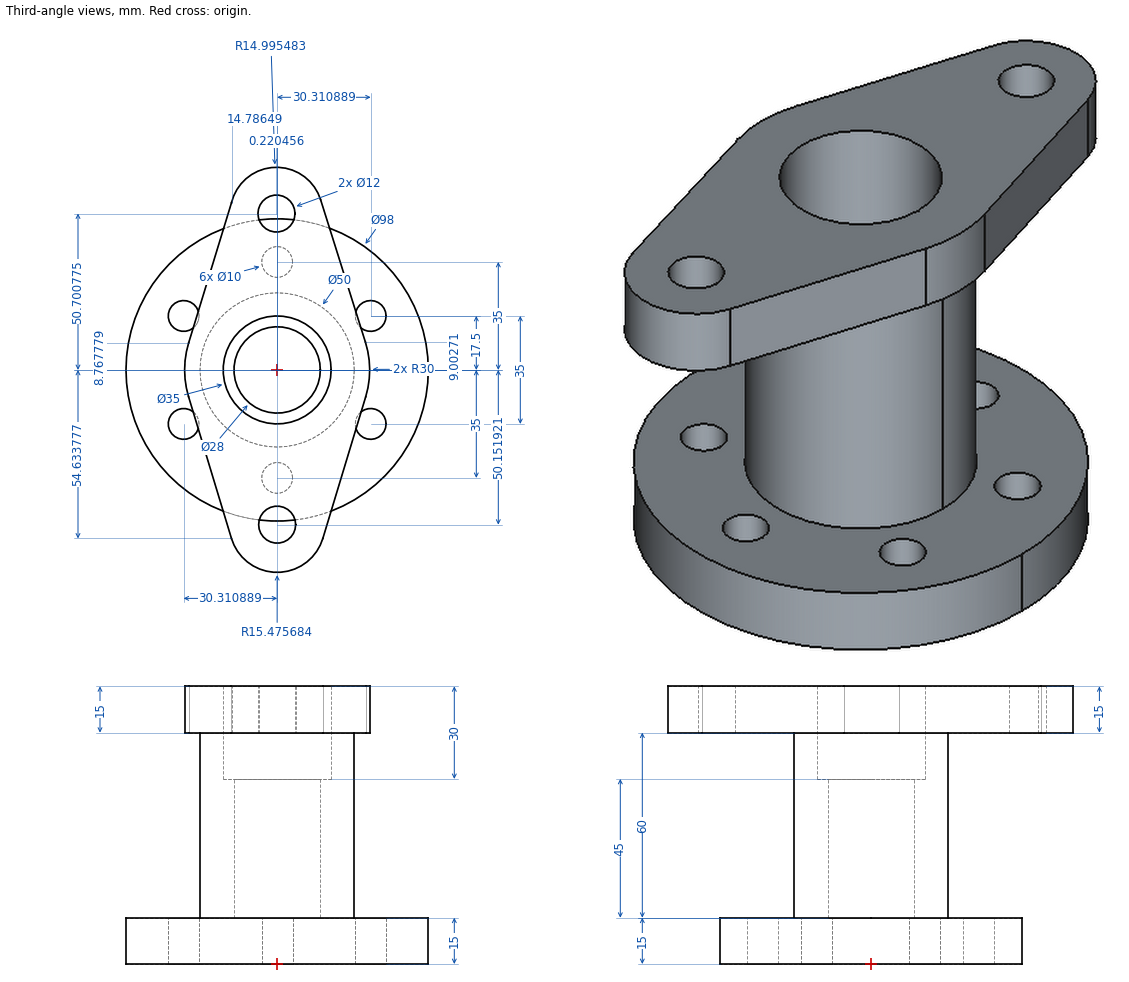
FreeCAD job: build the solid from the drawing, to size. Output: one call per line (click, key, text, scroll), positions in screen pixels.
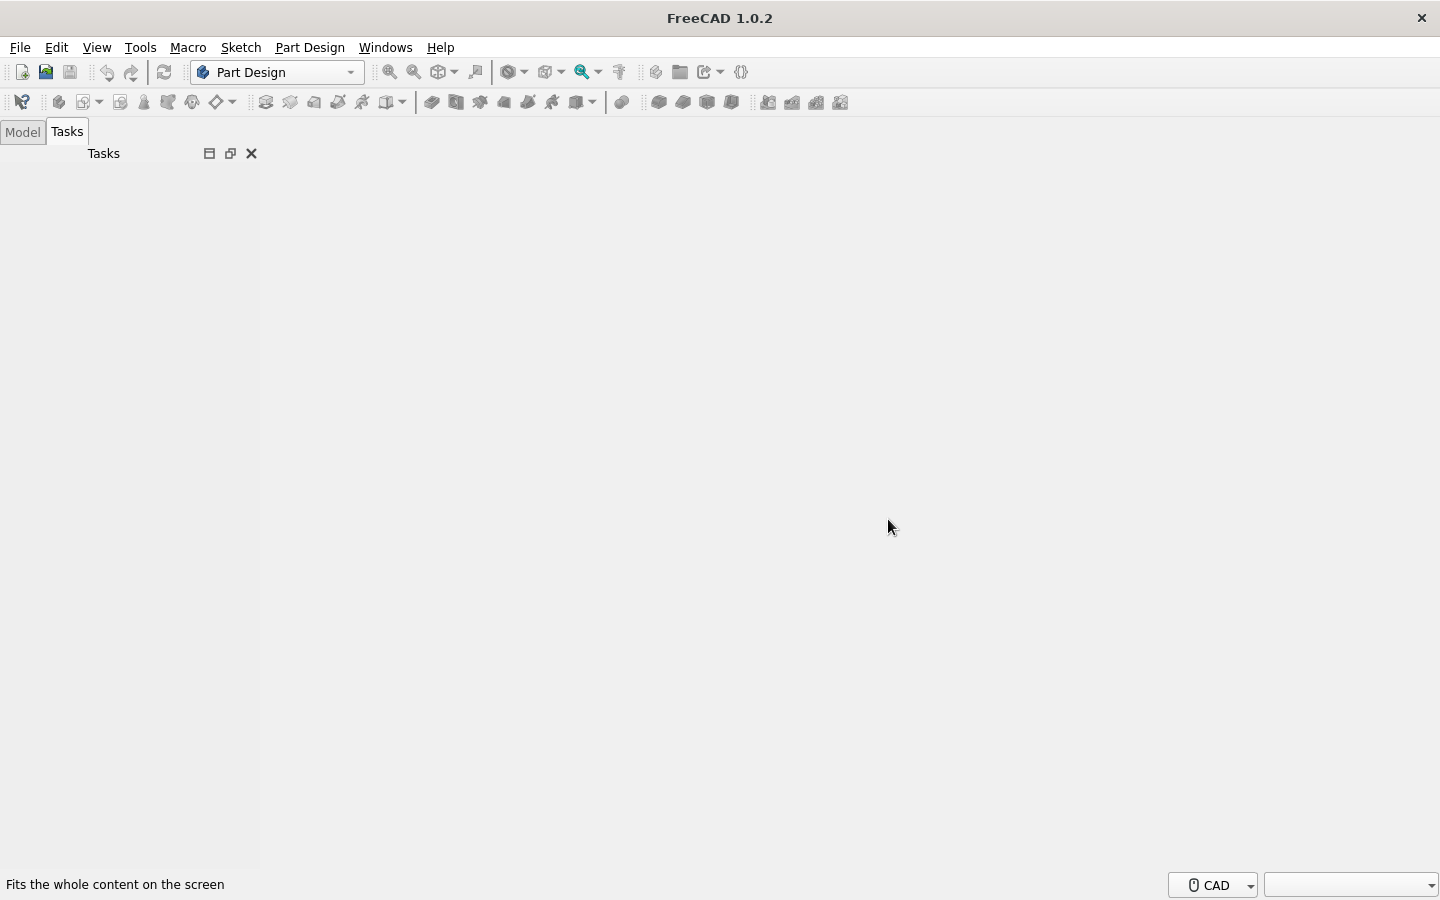
key(ctrl+n)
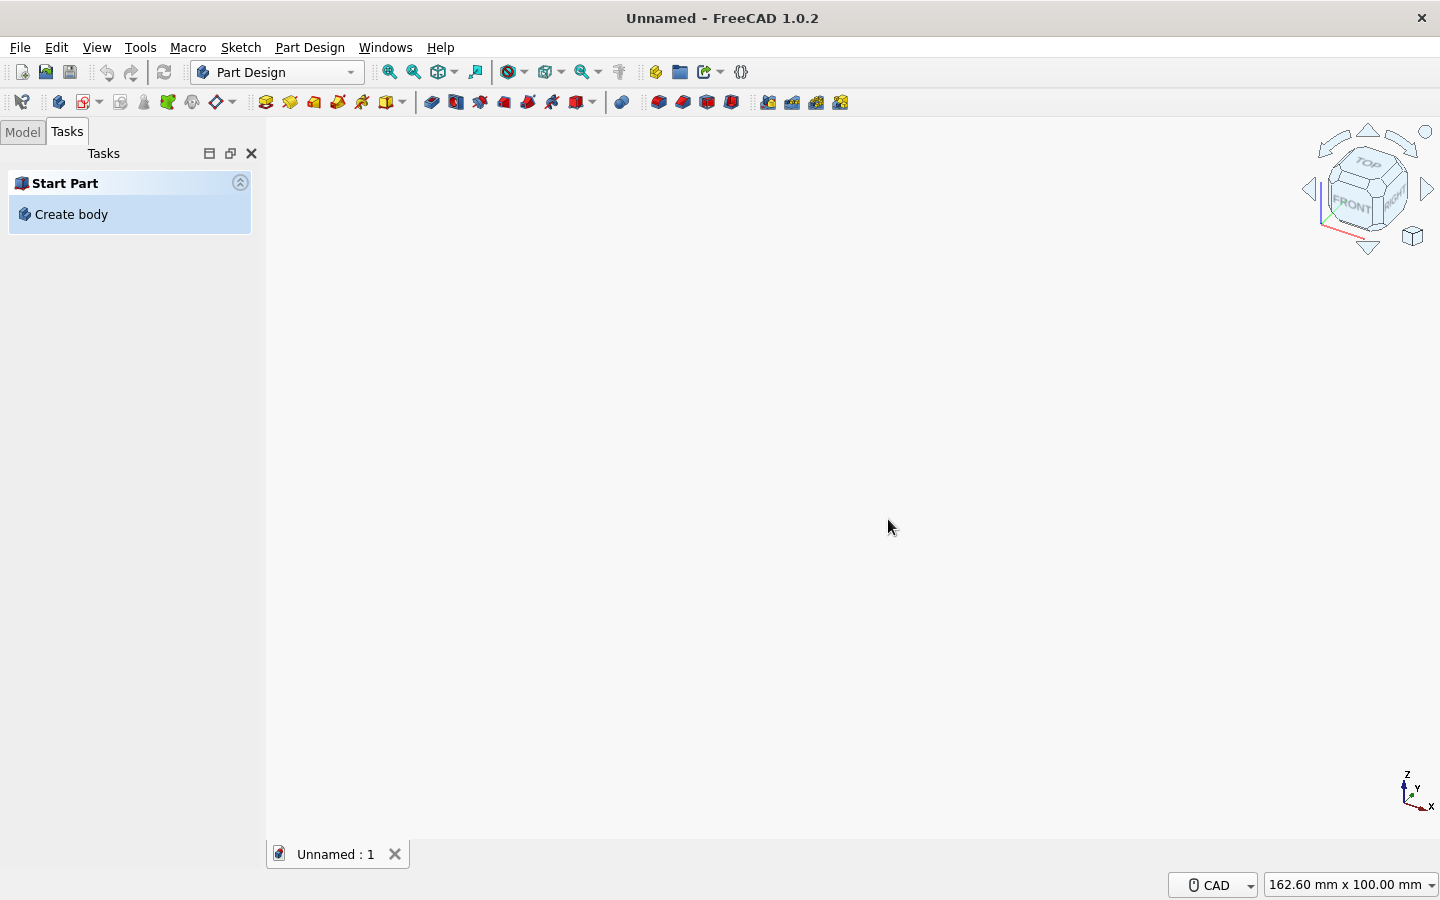
click(84, 102)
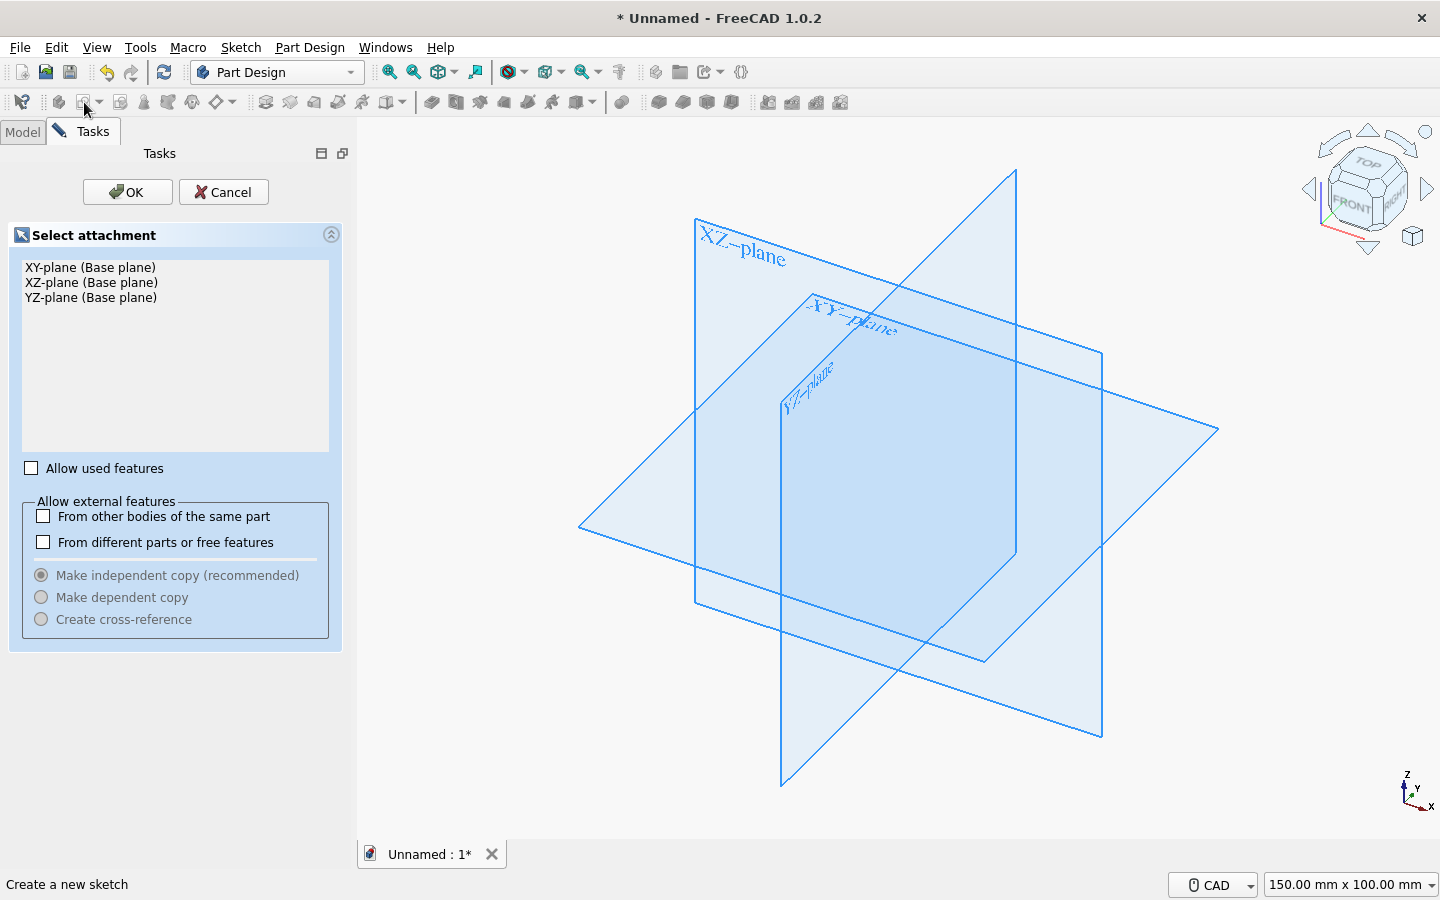
click(82, 268)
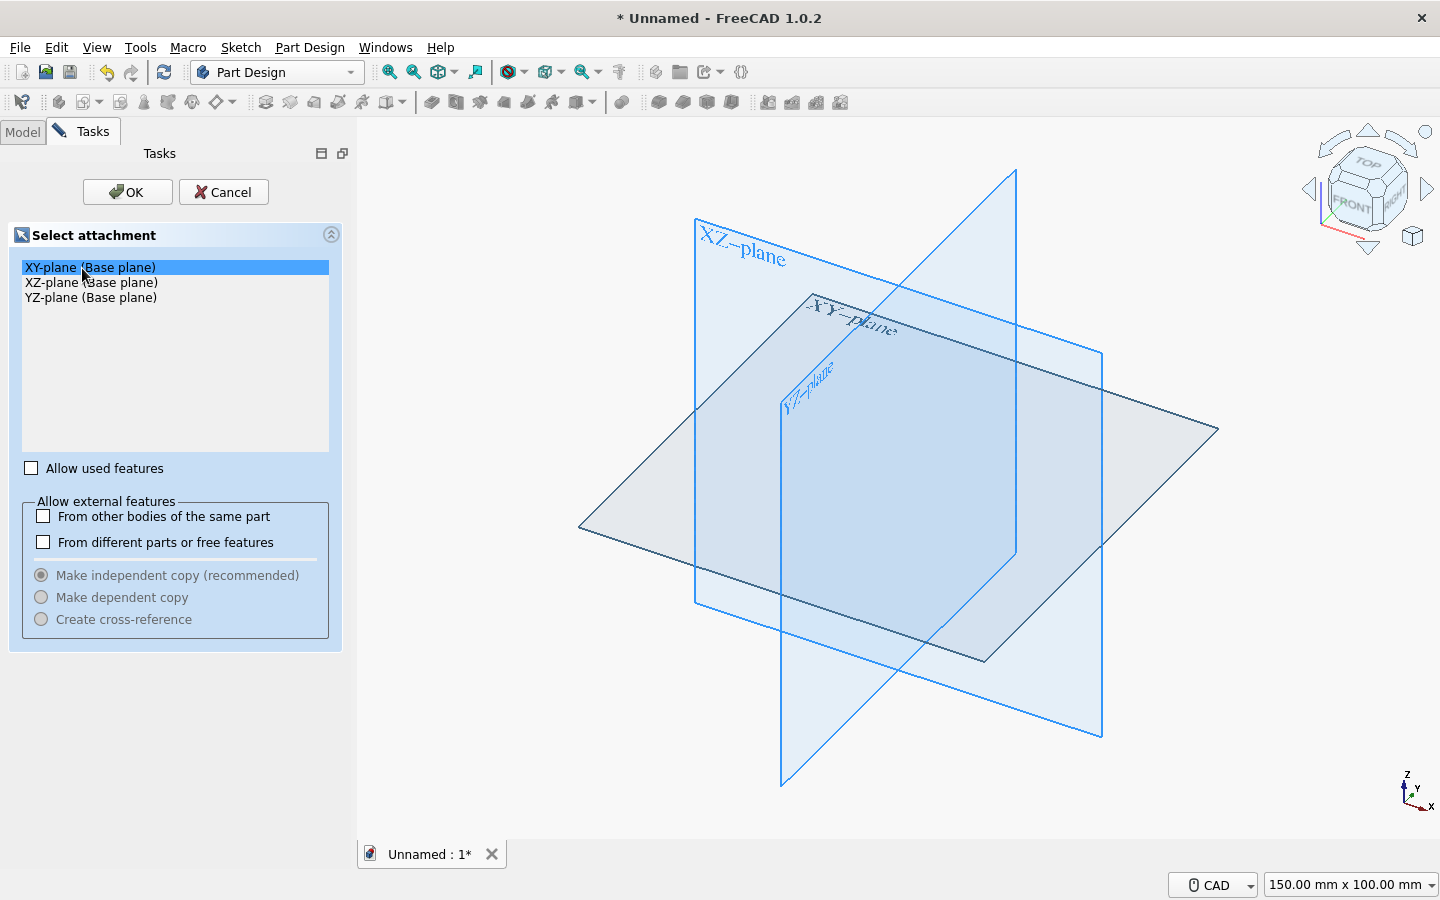
click(128, 192)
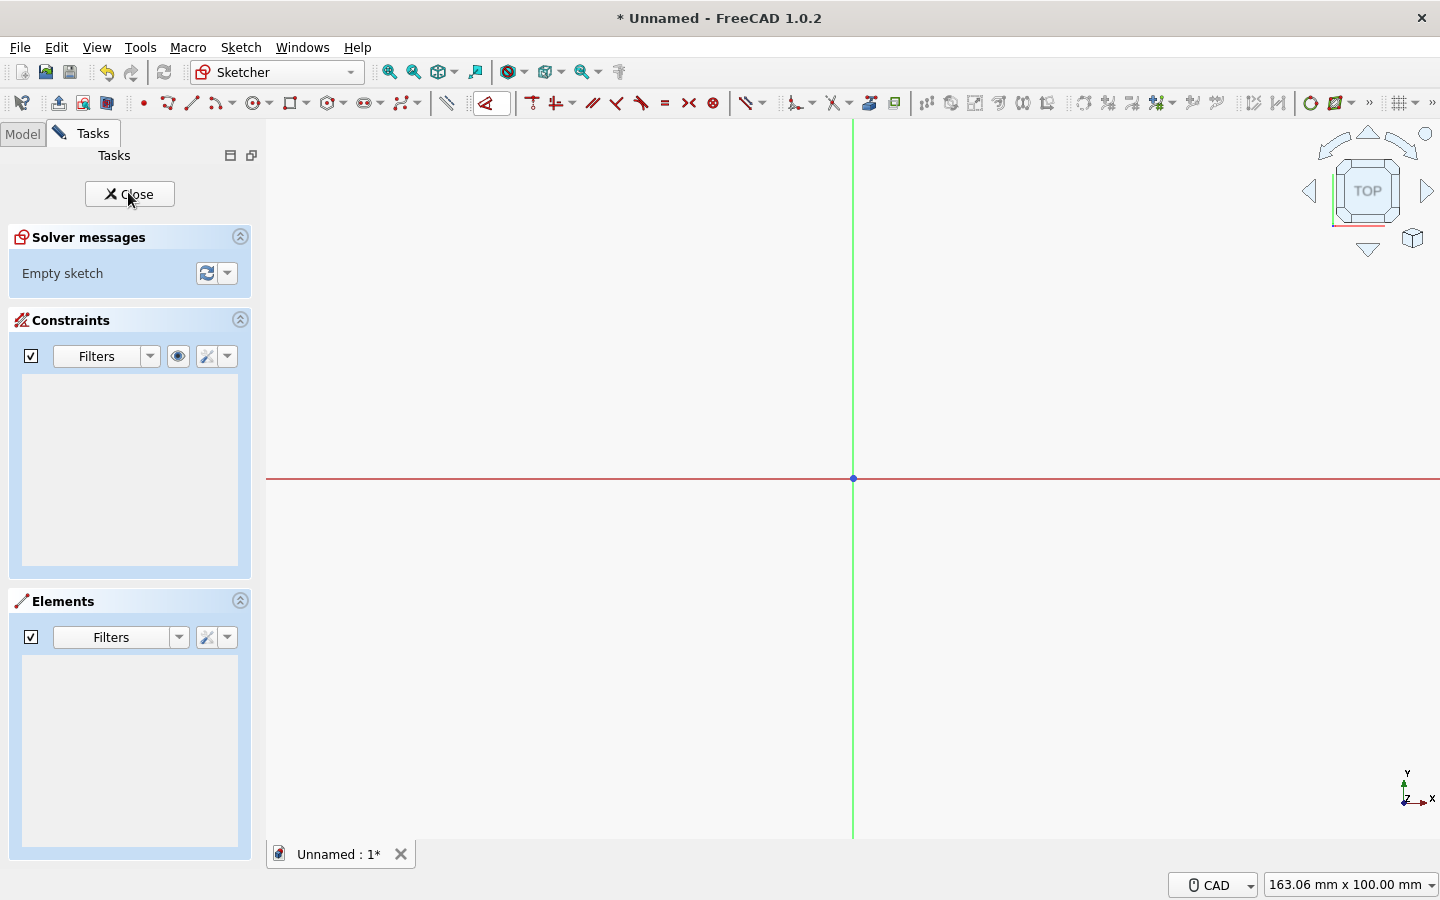
scroll(645, 479, down, 2)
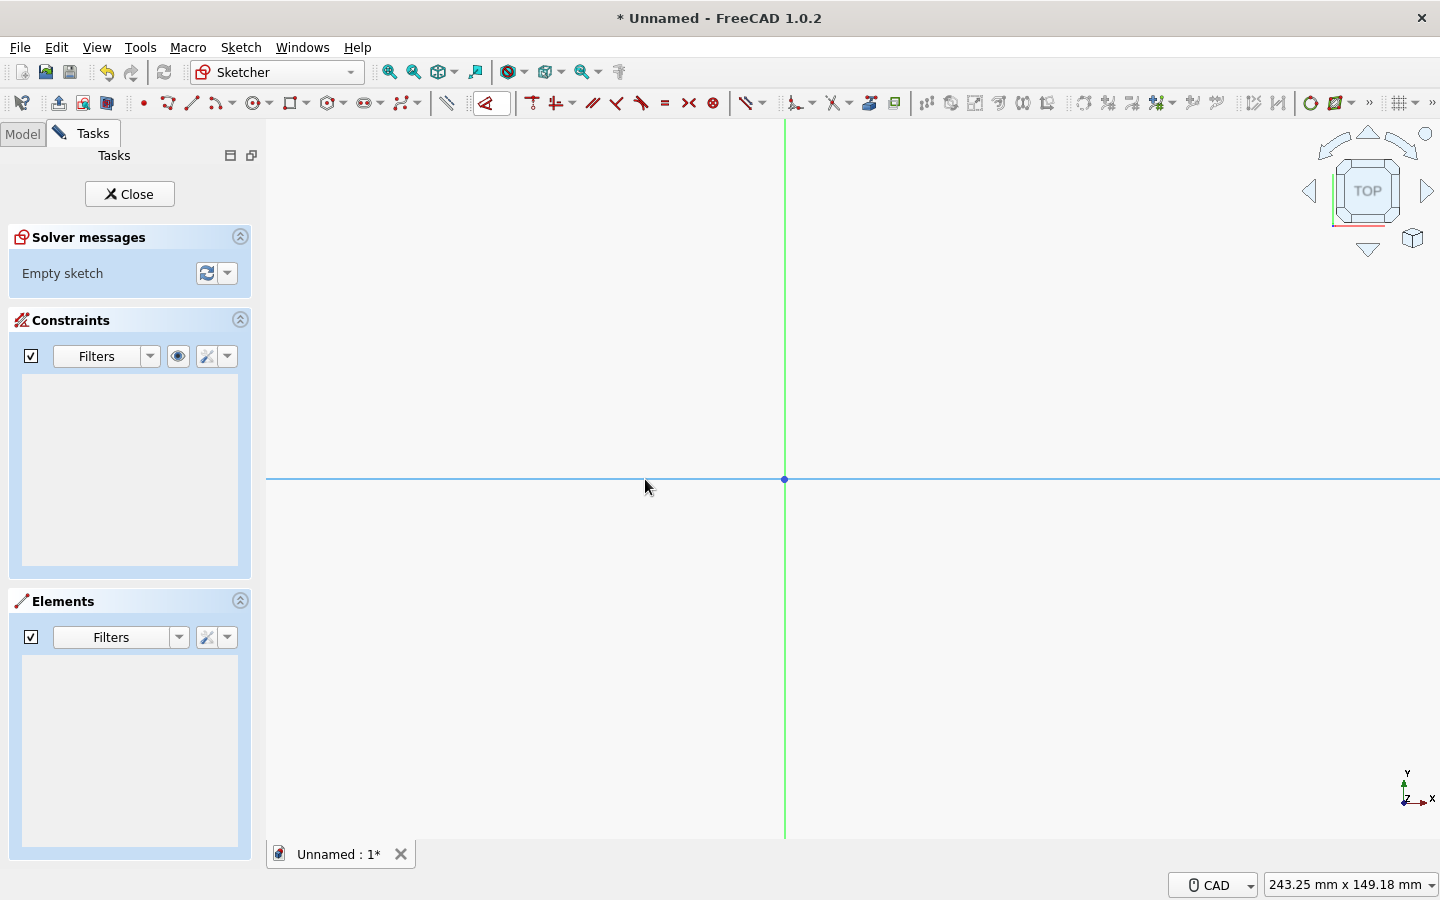
key(g)
key(c)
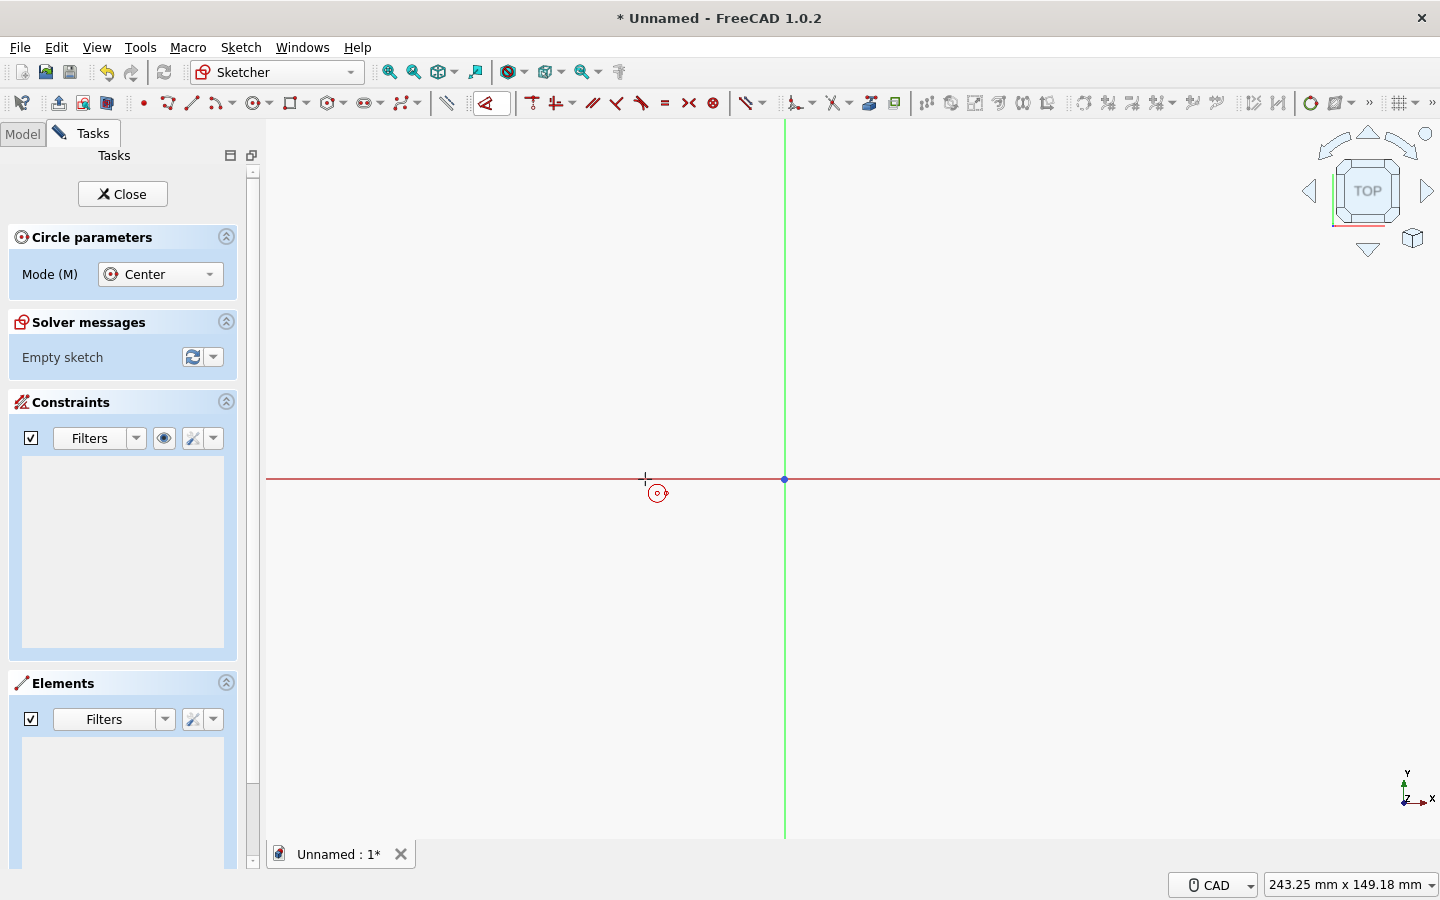
click(785, 479)
click(952, 312)
key(Escape)